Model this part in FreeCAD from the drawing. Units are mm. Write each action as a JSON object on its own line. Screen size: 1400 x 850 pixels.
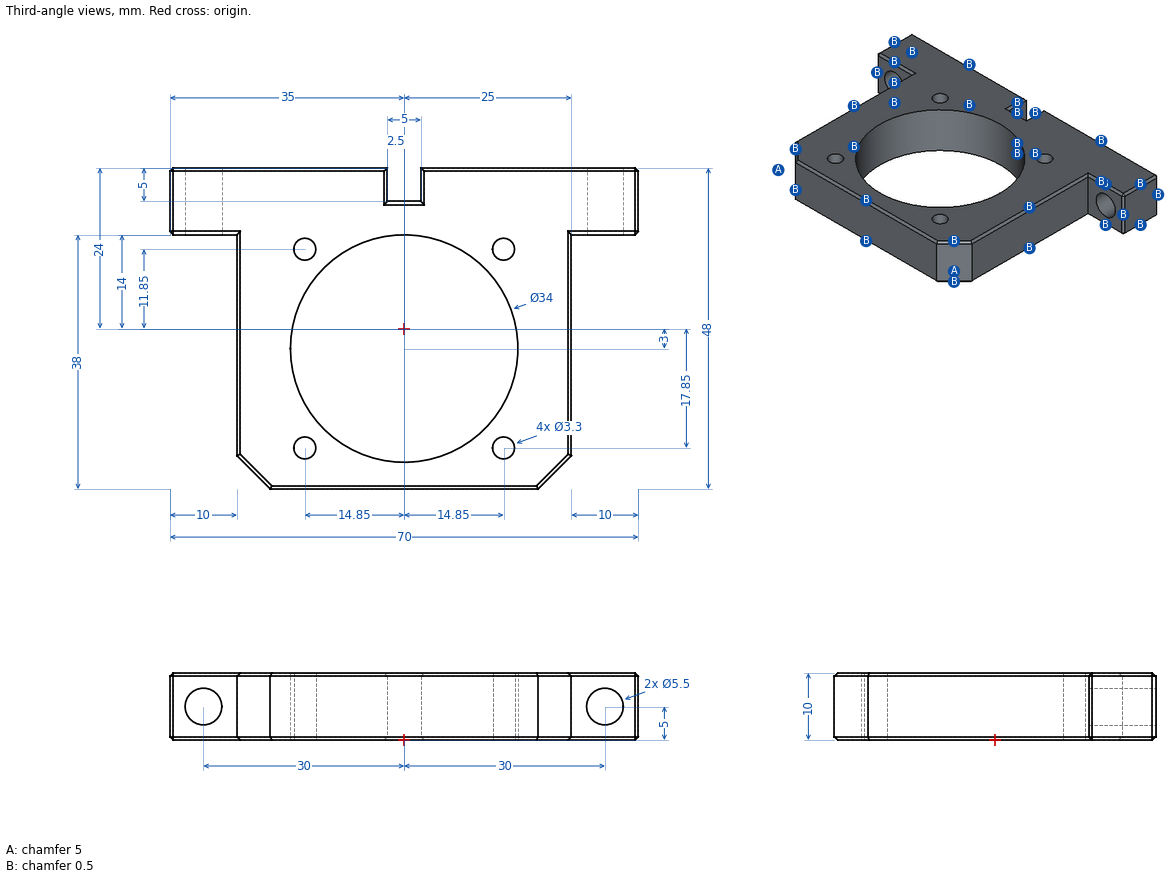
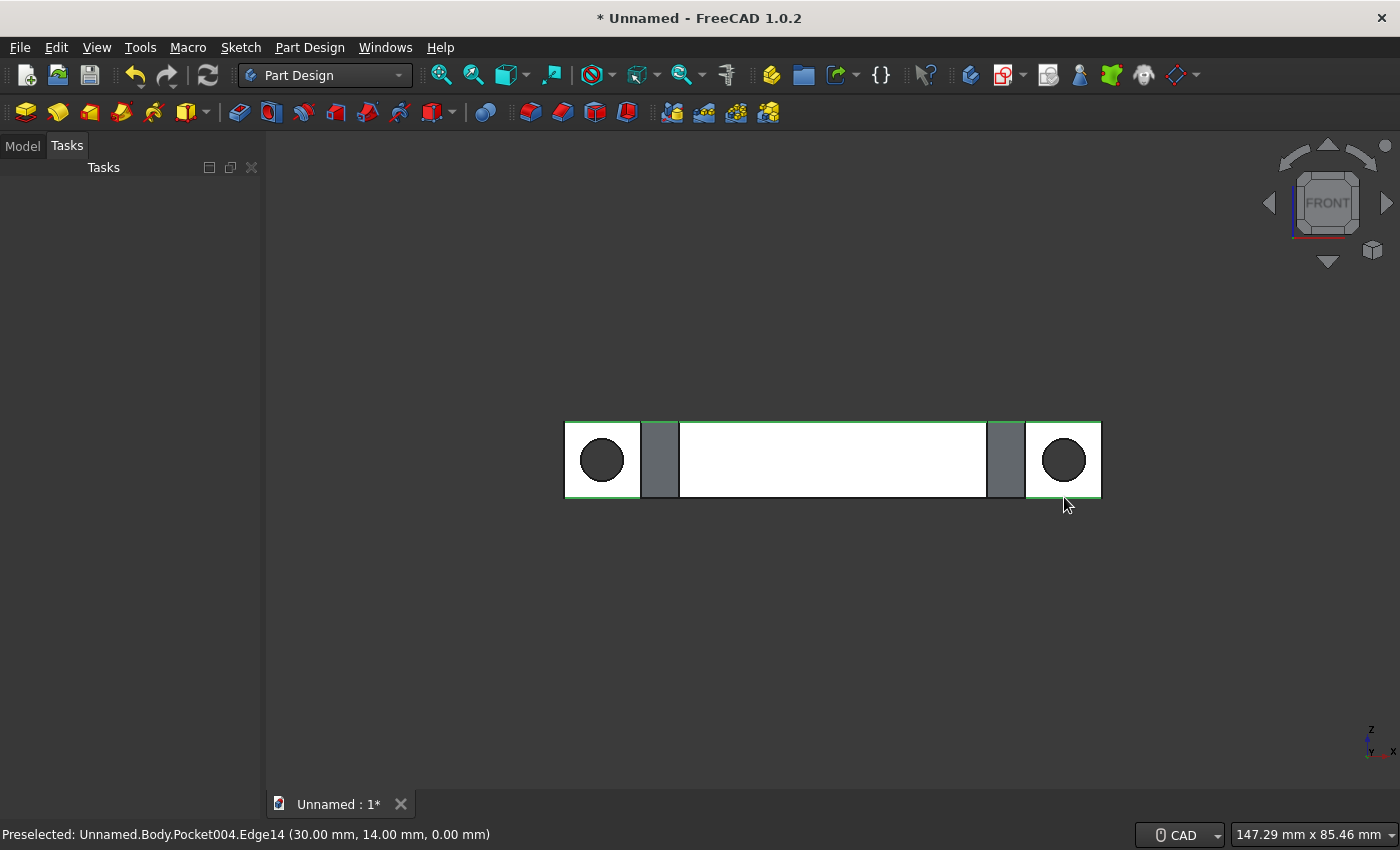
{"action": "left_click", "coordinate": [833, 497], "text": "ctrl"}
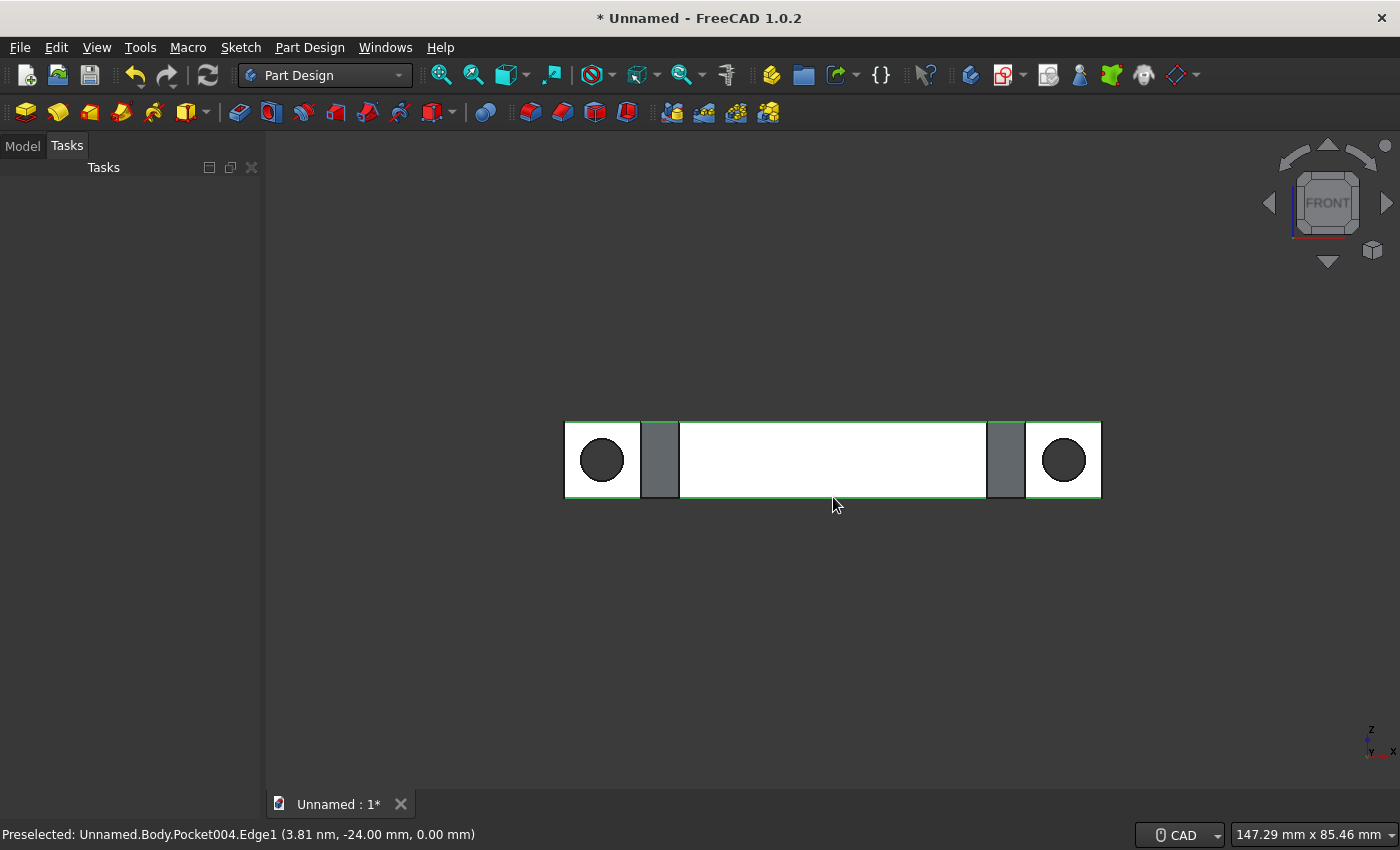
{"action": "left_click", "coordinate": [1006, 497], "text": "ctrl"}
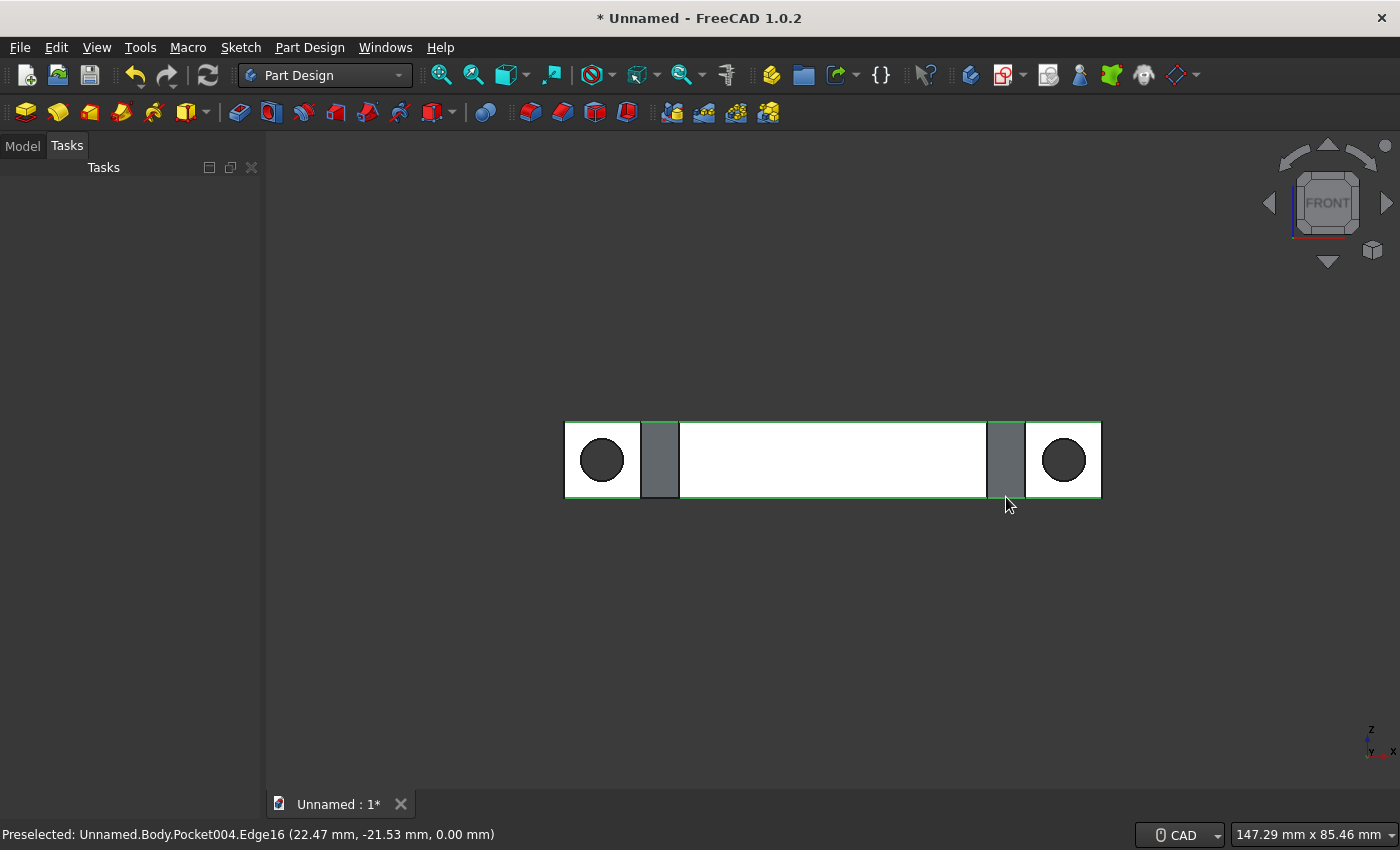
{"action": "left_click", "coordinate": [660, 497], "text": "ctrl"}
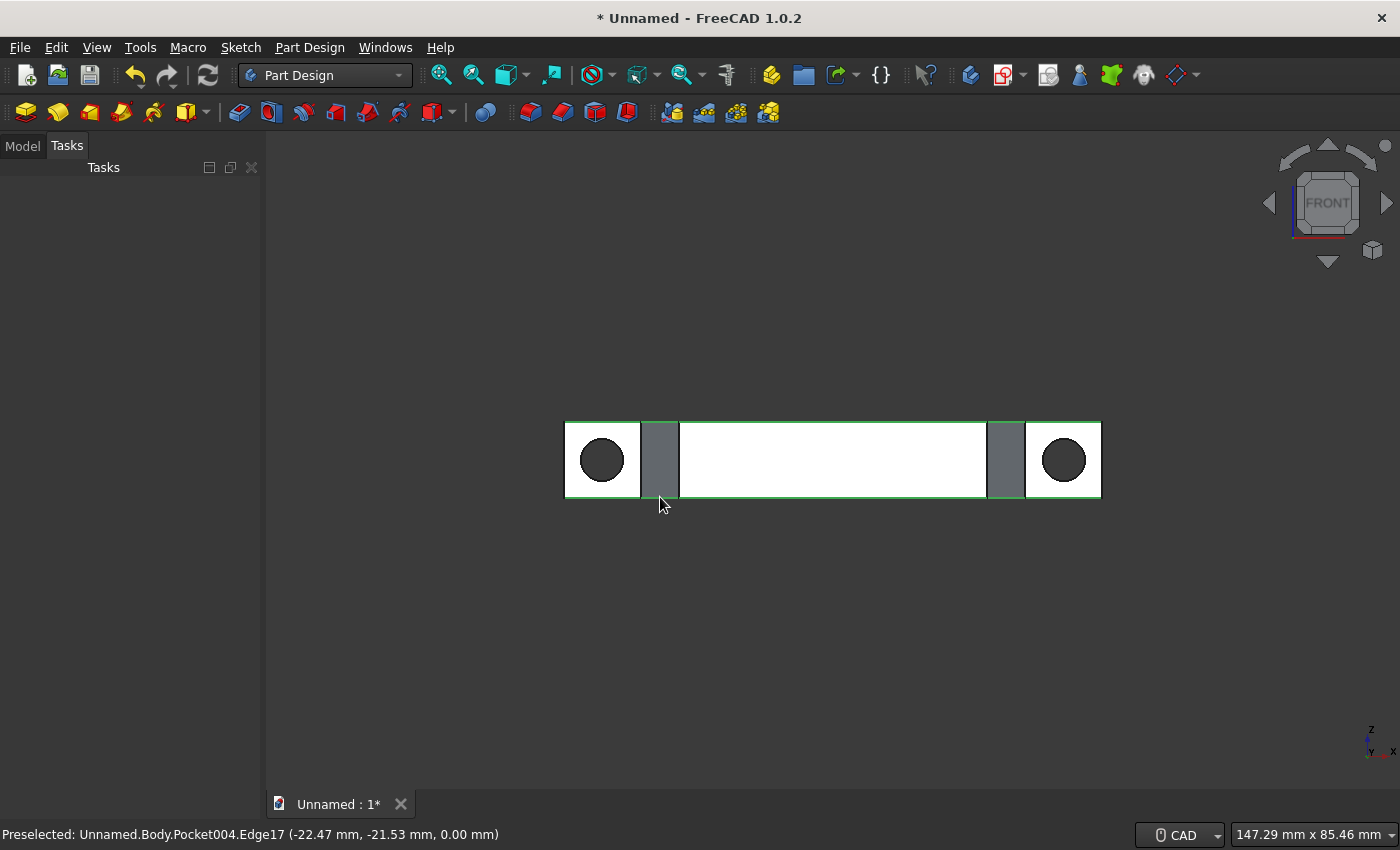
{"action": "key", "text": "3"}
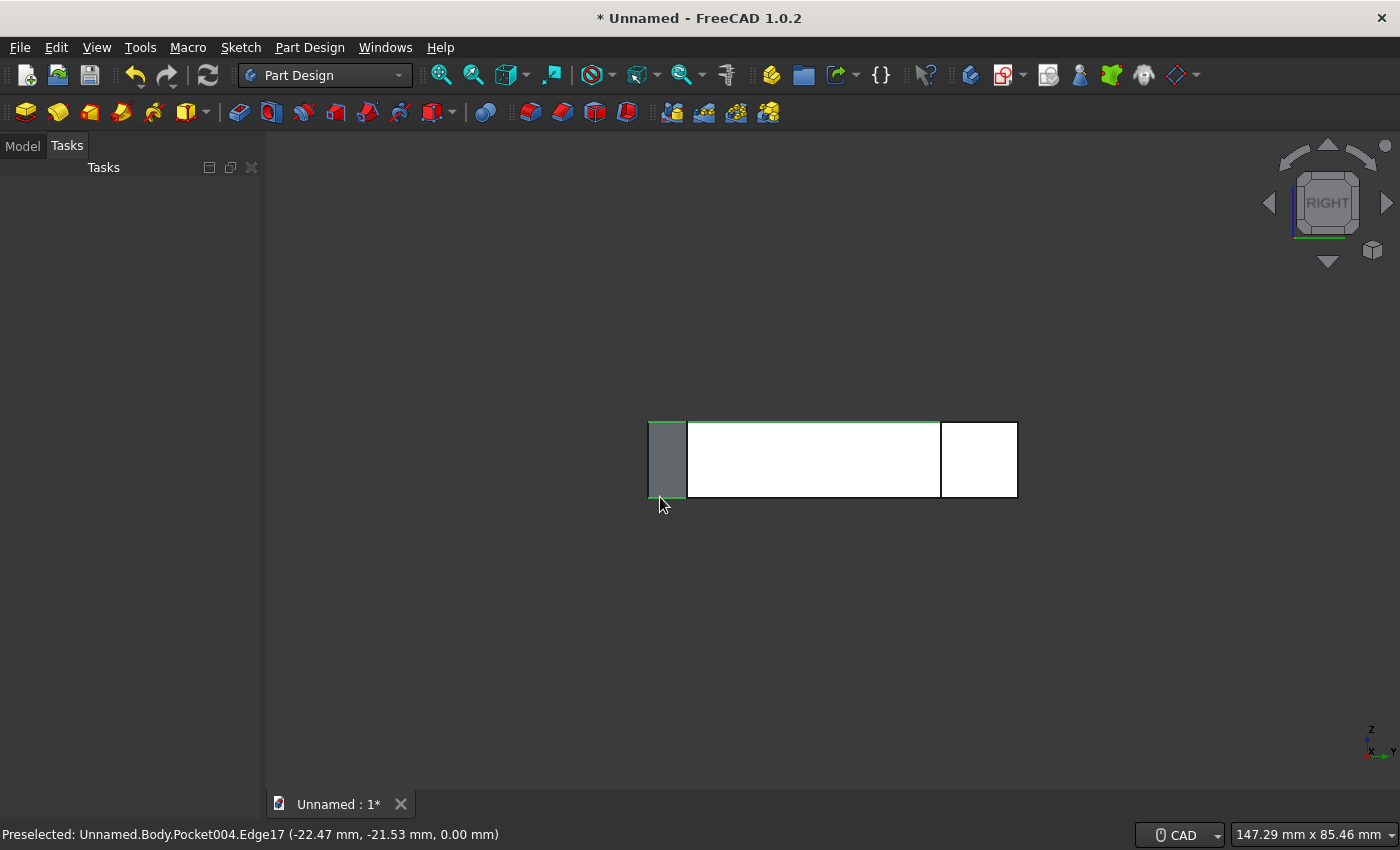
{"action": "left_click", "coordinate": [442, 76]}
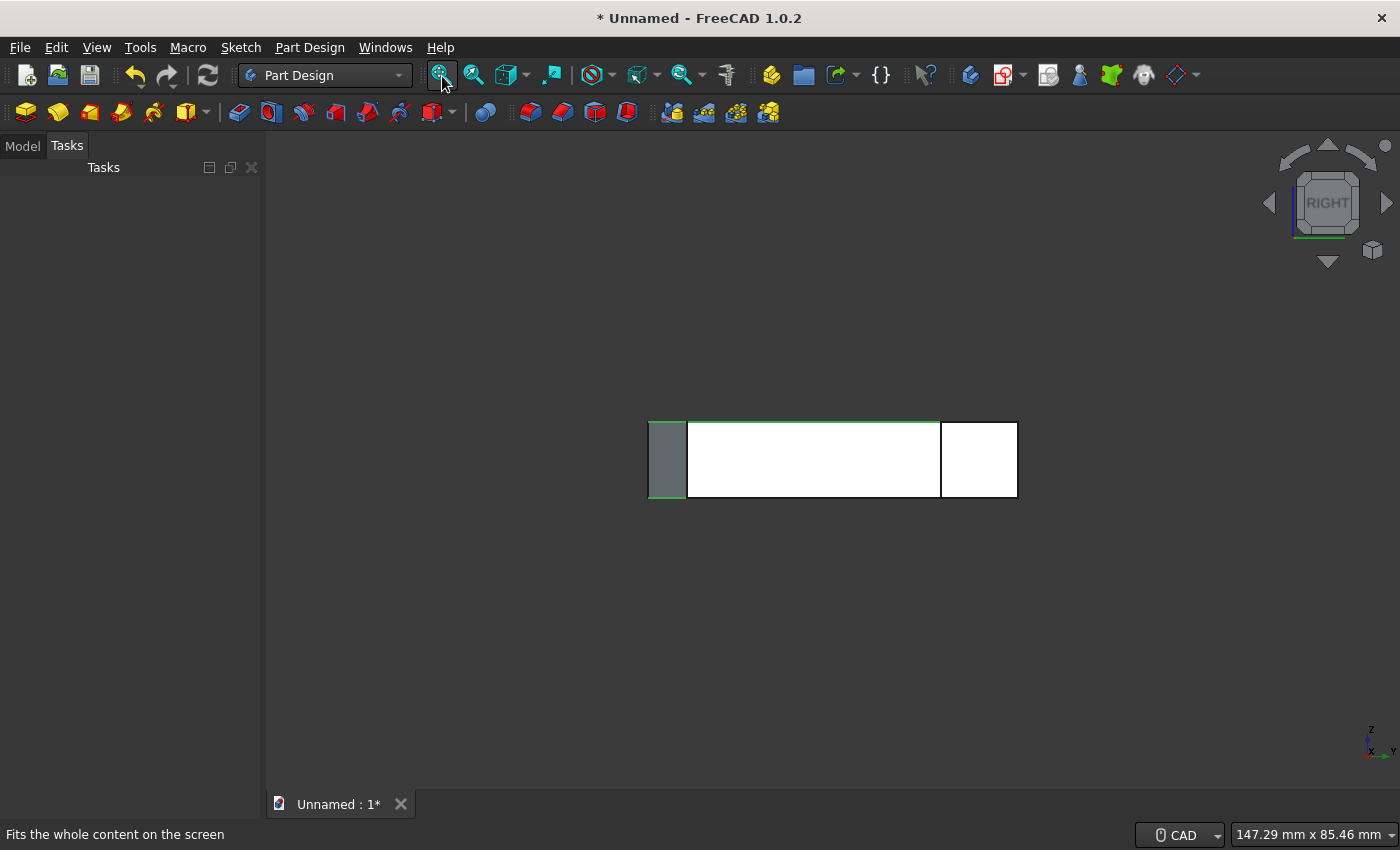
{"action": "left_click", "coordinate": [814, 497], "text": "ctrl"}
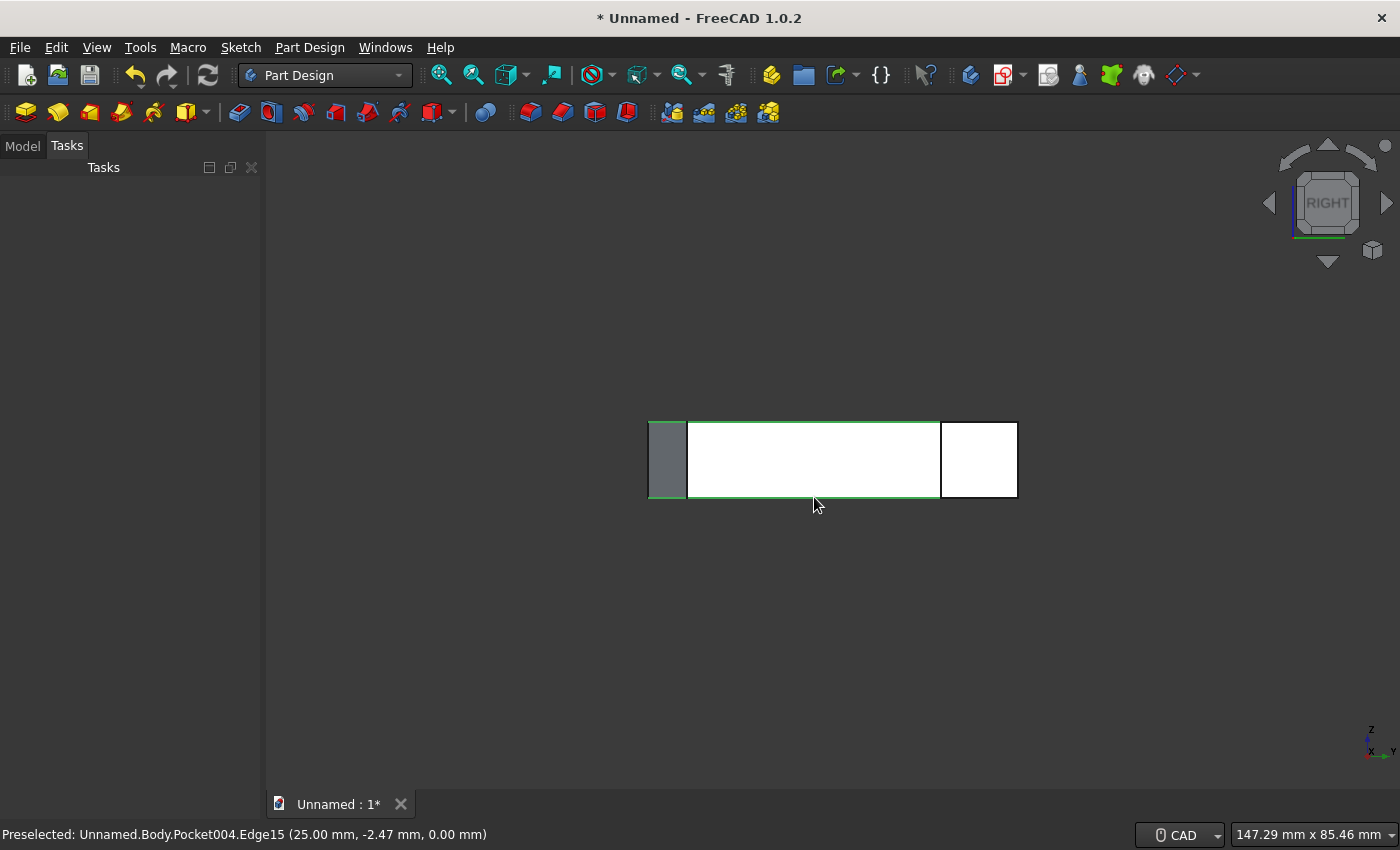
{"action": "key", "text": "5"}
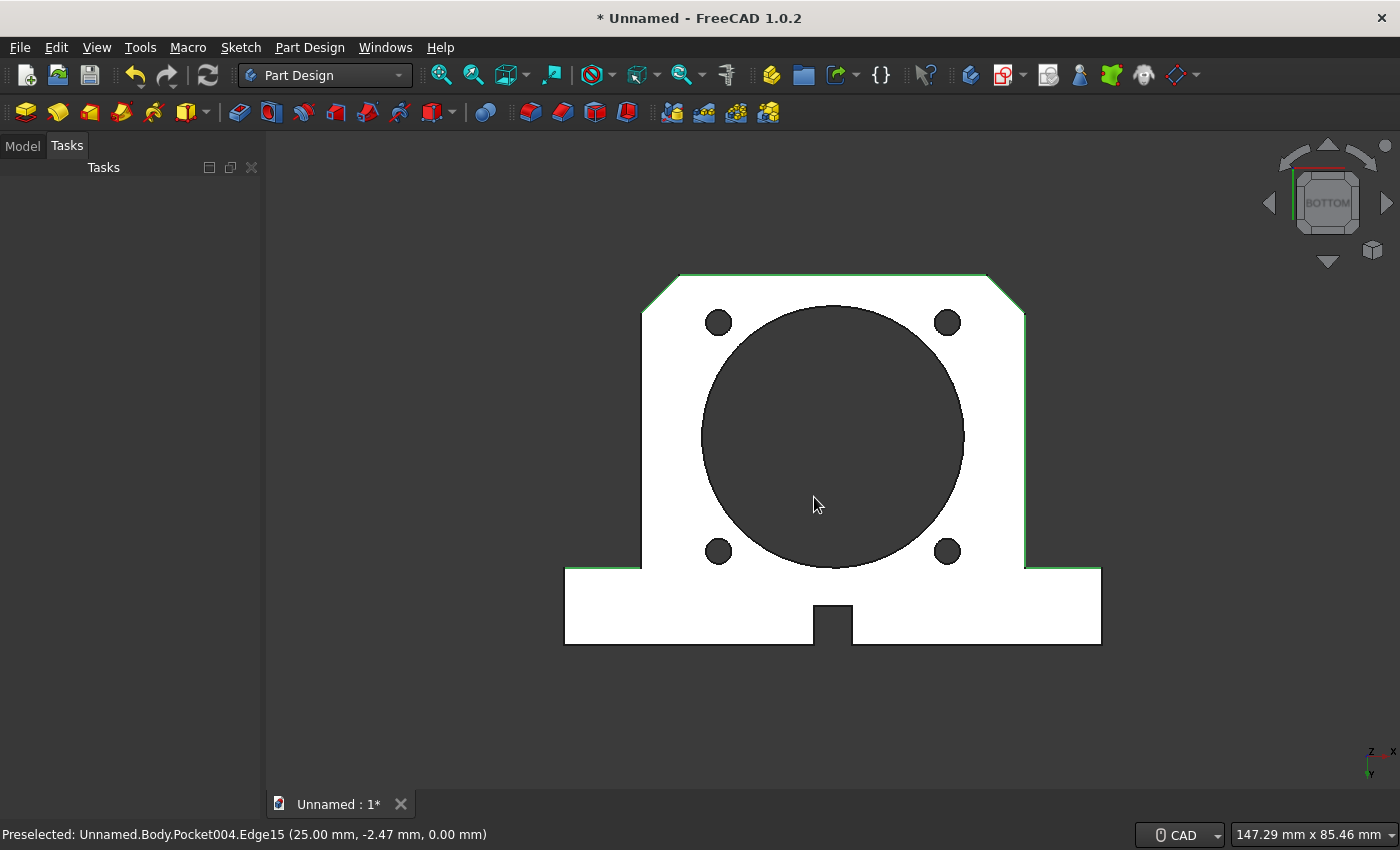
{"action": "left_click", "coordinate": [977, 644], "text": "ctrl"}